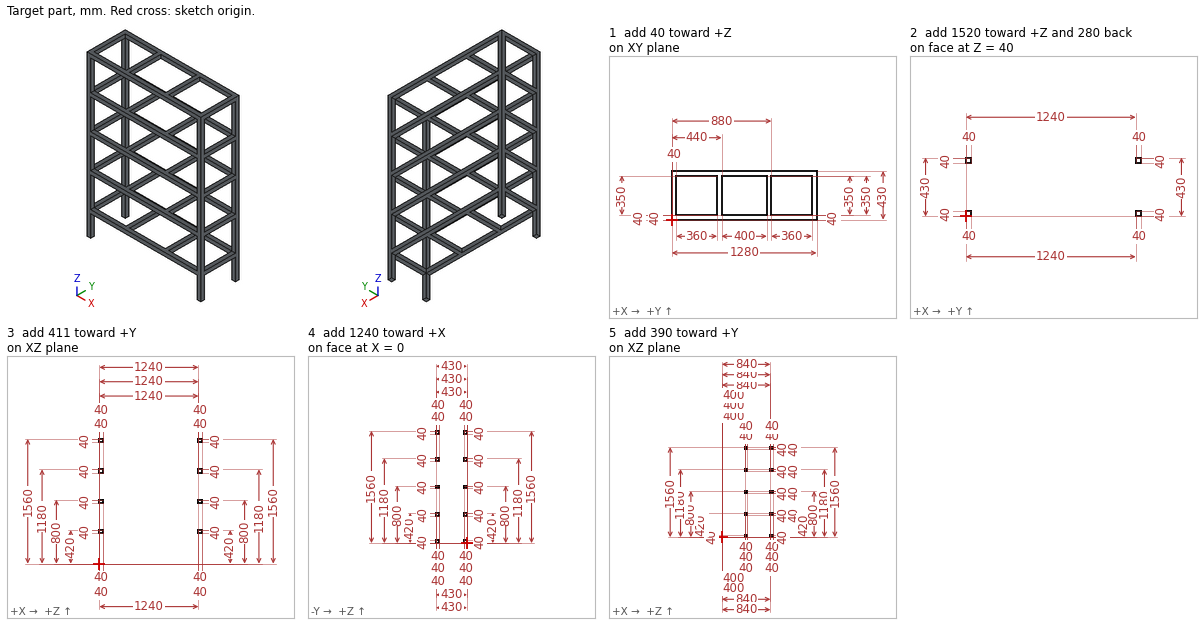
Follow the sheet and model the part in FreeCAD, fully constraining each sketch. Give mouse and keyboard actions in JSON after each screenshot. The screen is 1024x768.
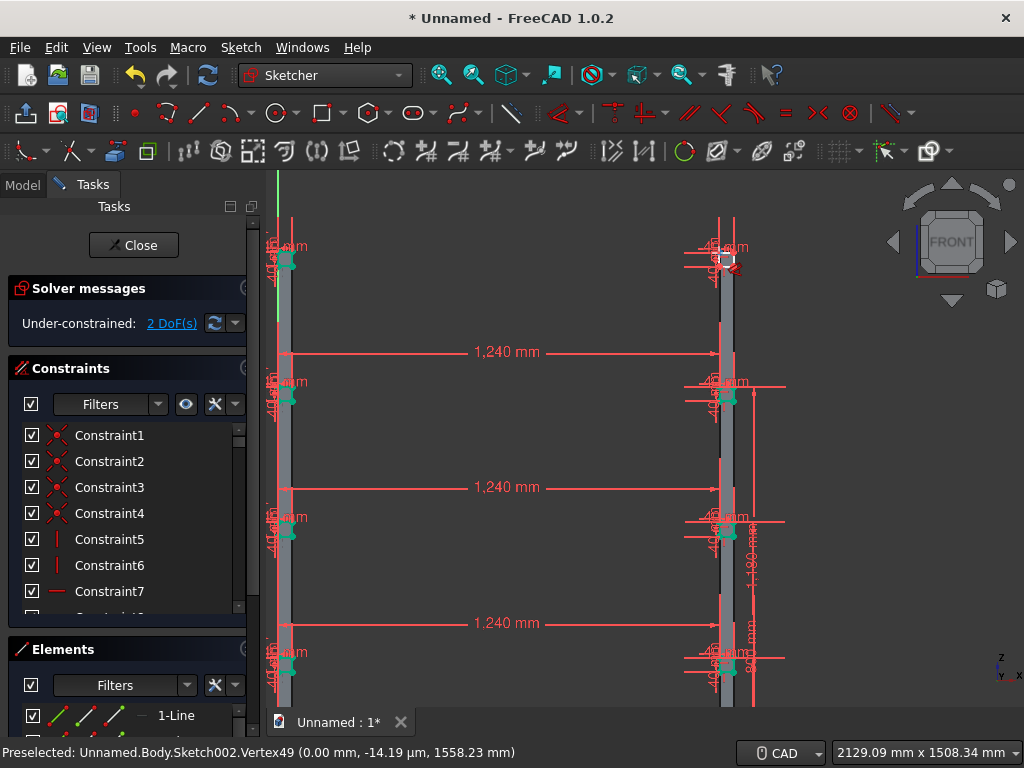
{"action": "left_click", "coordinate": [719, 253]}
{"action": "left_click", "coordinate": [507, 219]}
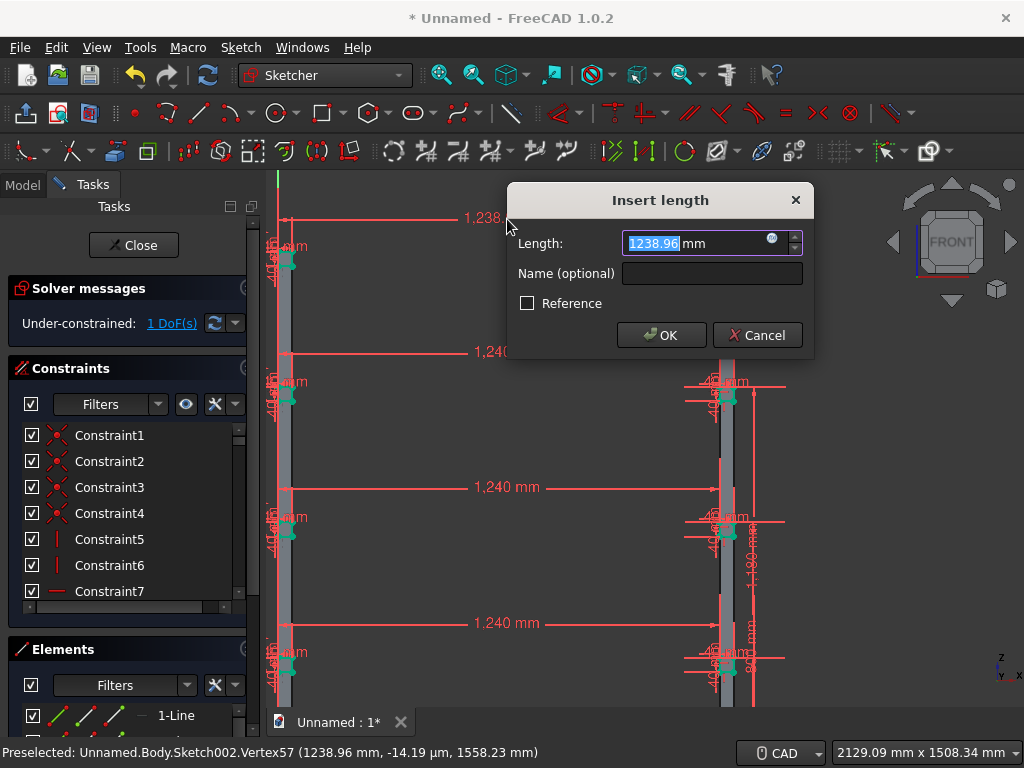
{"action": "type", "text": "1240"}
{"action": "key", "text": "Return"}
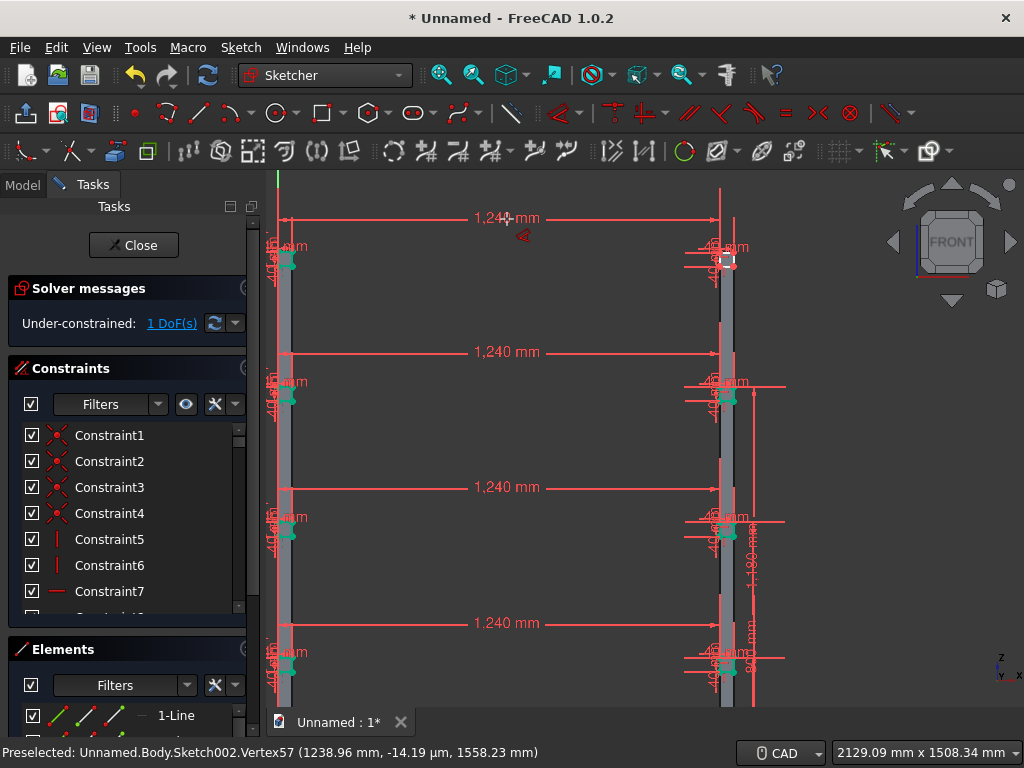
{"action": "left_click", "coordinate": [720, 253]}
{"action": "left_click", "coordinate": [754, 466]}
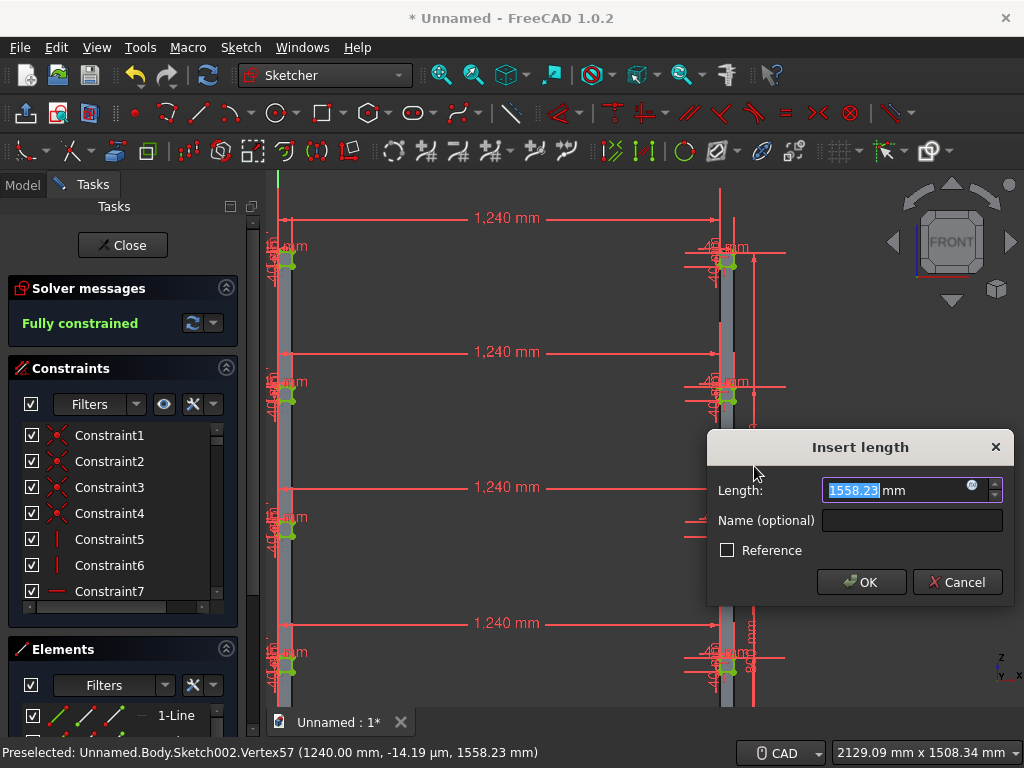
{"action": "type", "text": "1560"}
{"action": "key", "text": "Return"}
{"action": "key", "text": "Escape"}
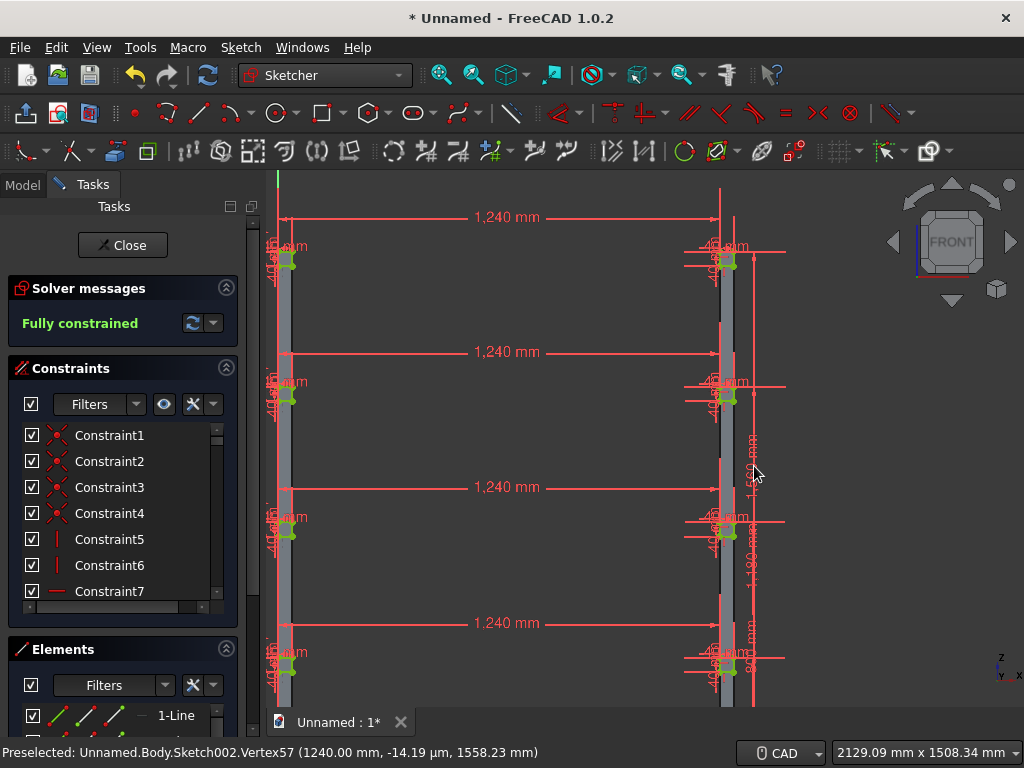
{"action": "left_click", "coordinate": [123, 245]}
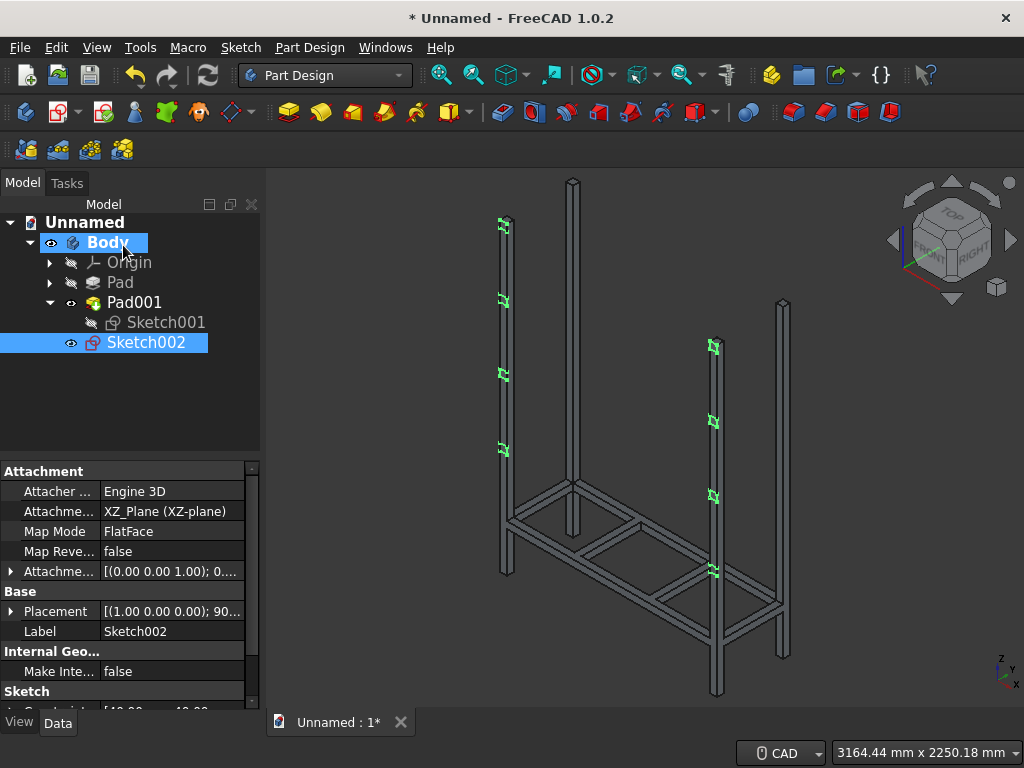
{"action": "left_click", "coordinate": [290, 112]}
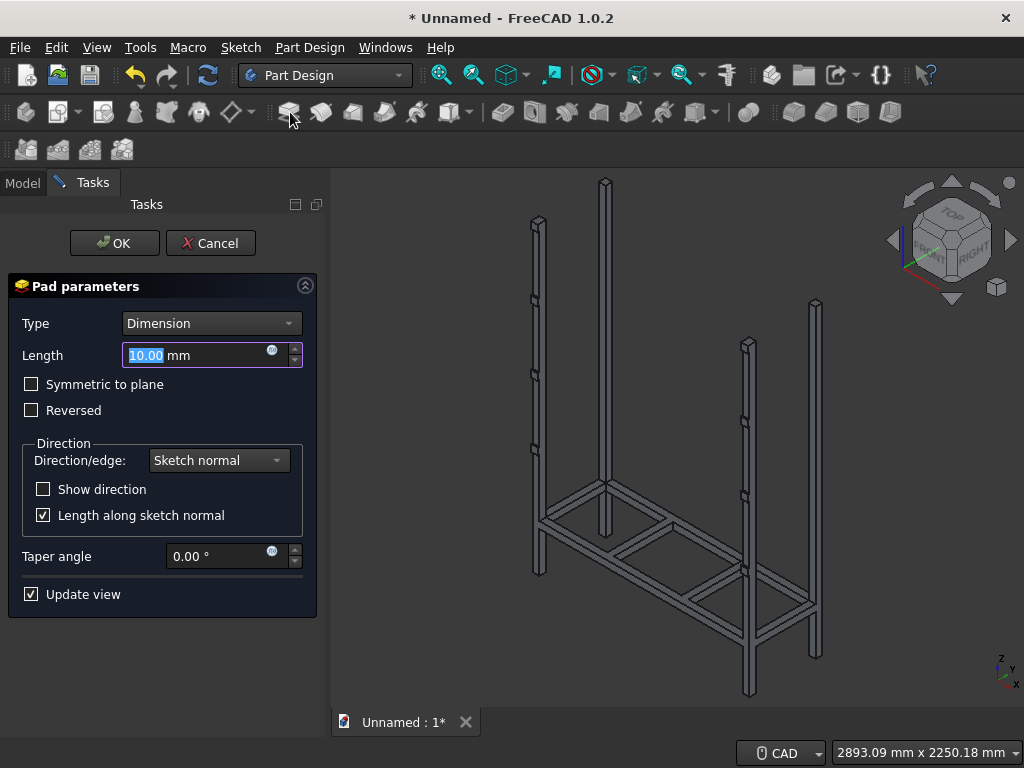
{"action": "type", "text": "411"}
{"action": "key", "text": "Tab"}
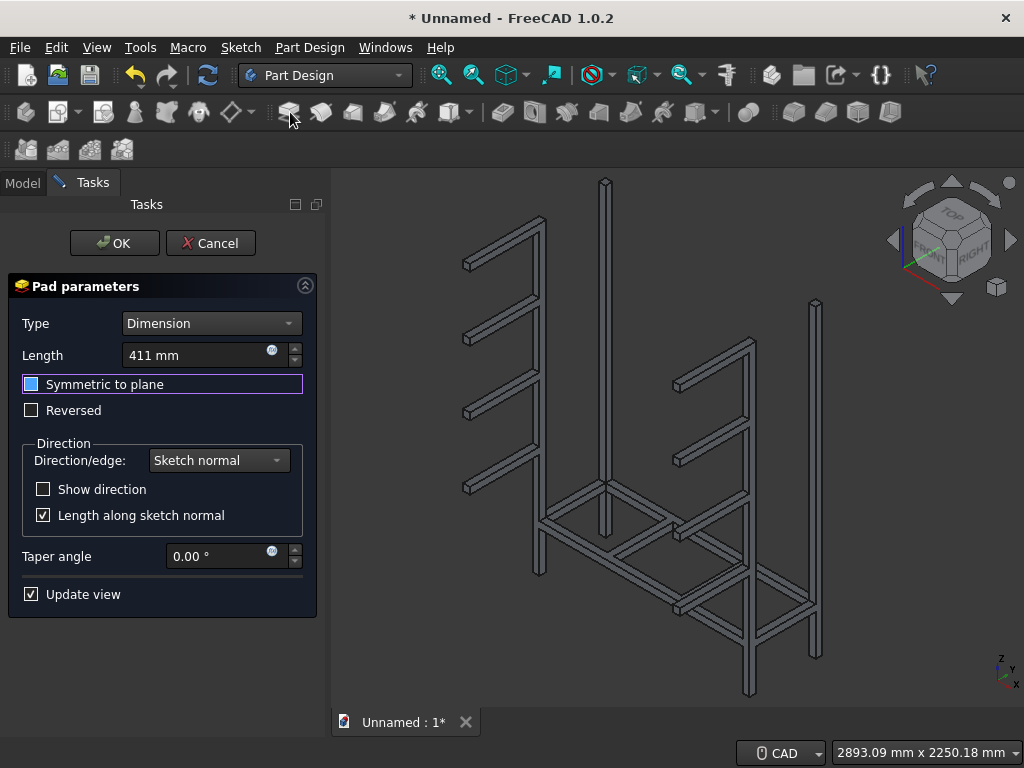
{"action": "left_click", "coordinate": [30, 410]}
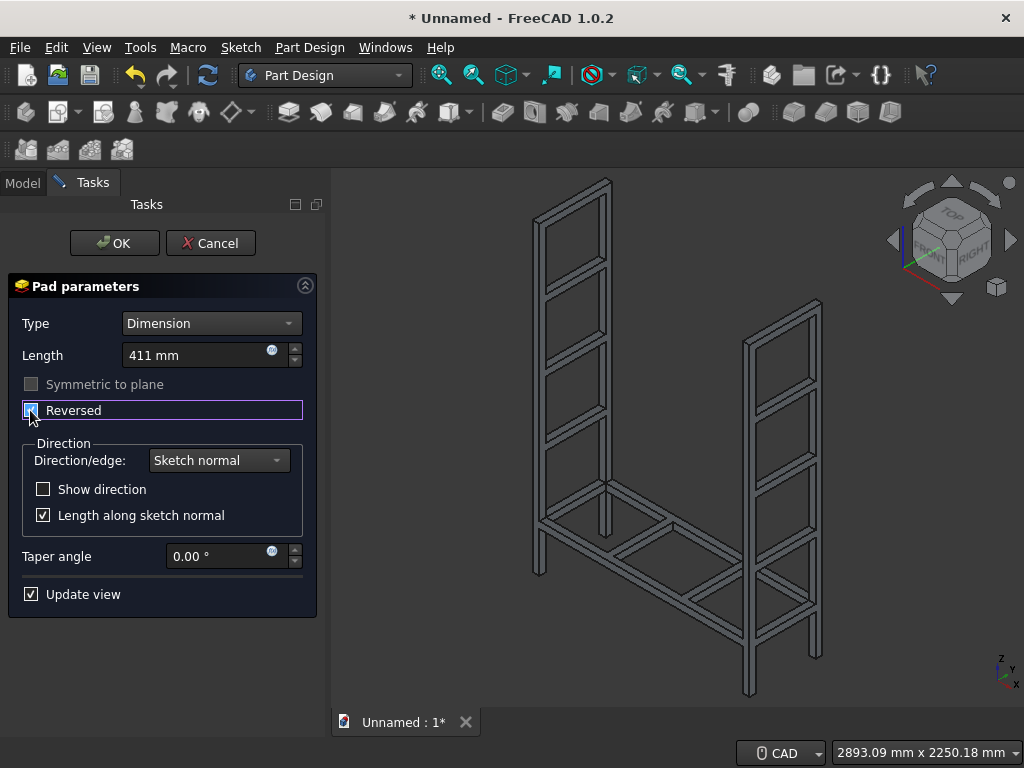
{"action": "left_click", "coordinate": [115, 243]}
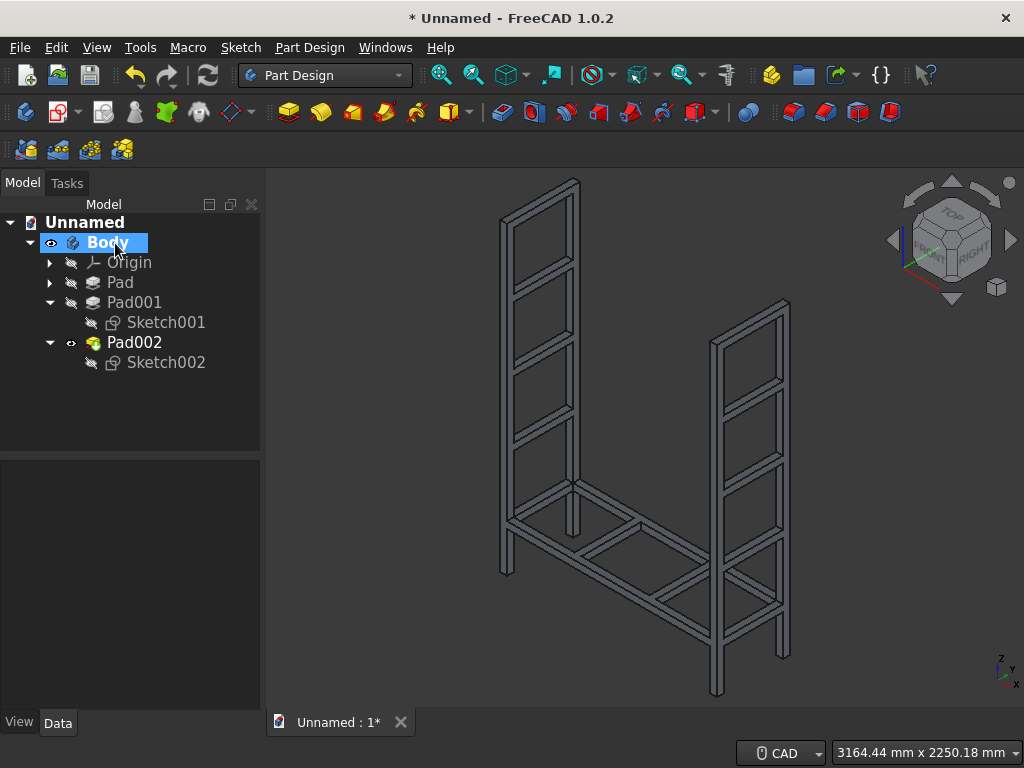
{"action": "key", "text": "6"}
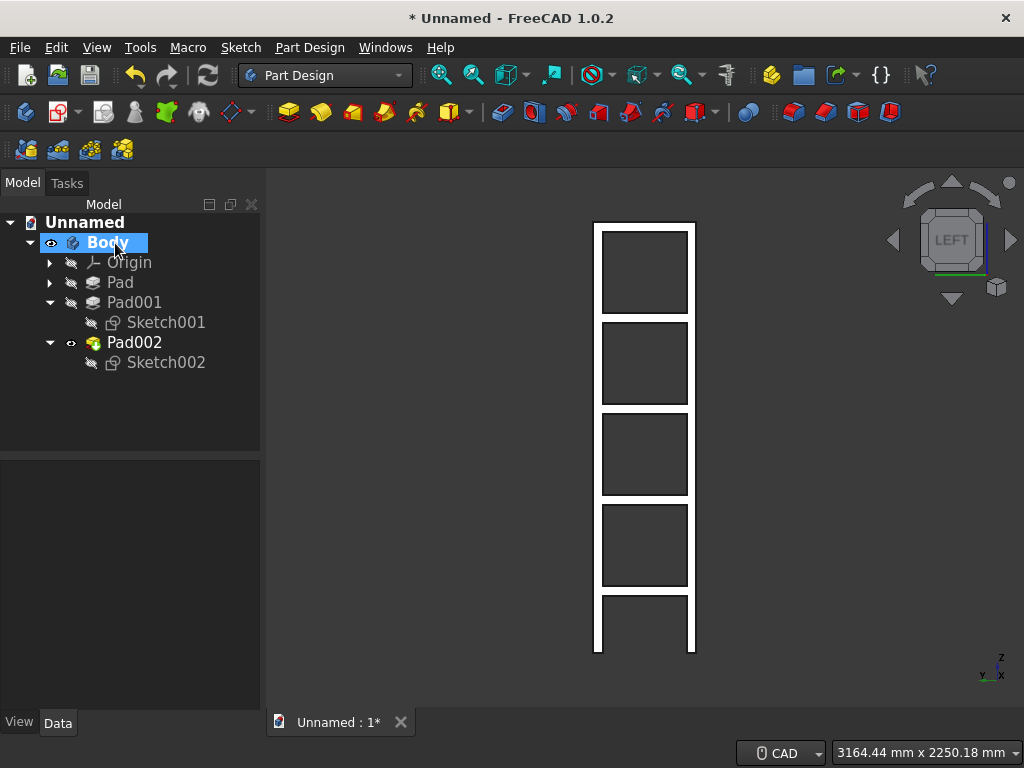
{"action": "scroll", "coordinate": [689, 498], "scroll_direction": "up", "scroll_amount": 5}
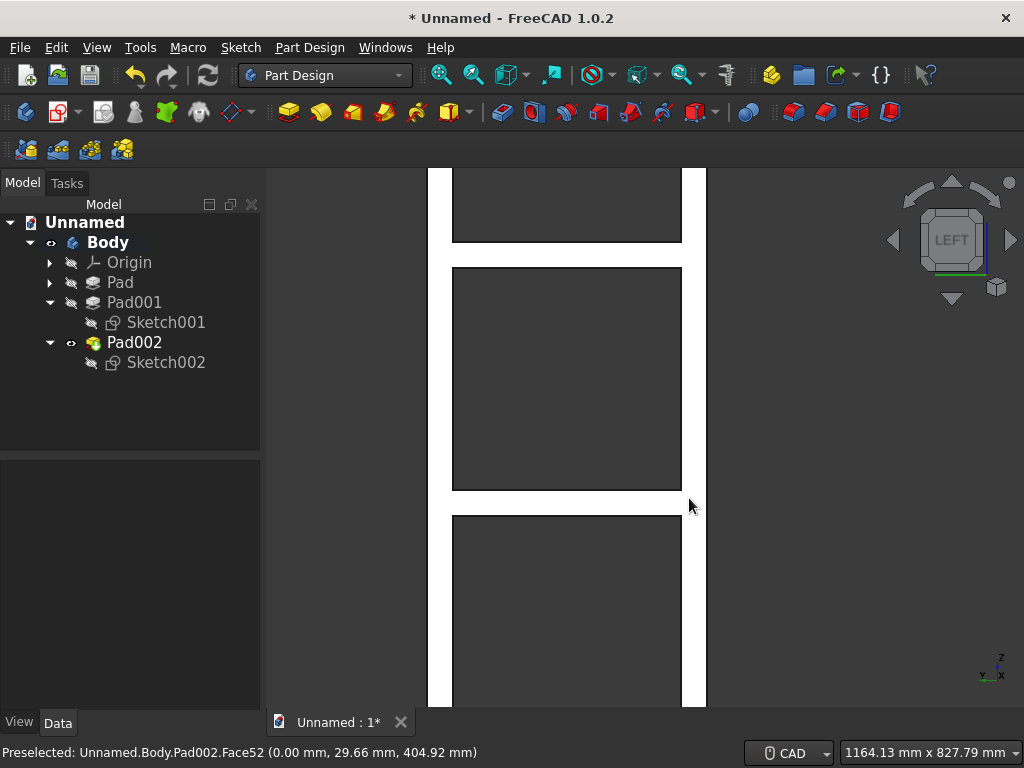
{"action": "left_click", "coordinate": [687, 500]}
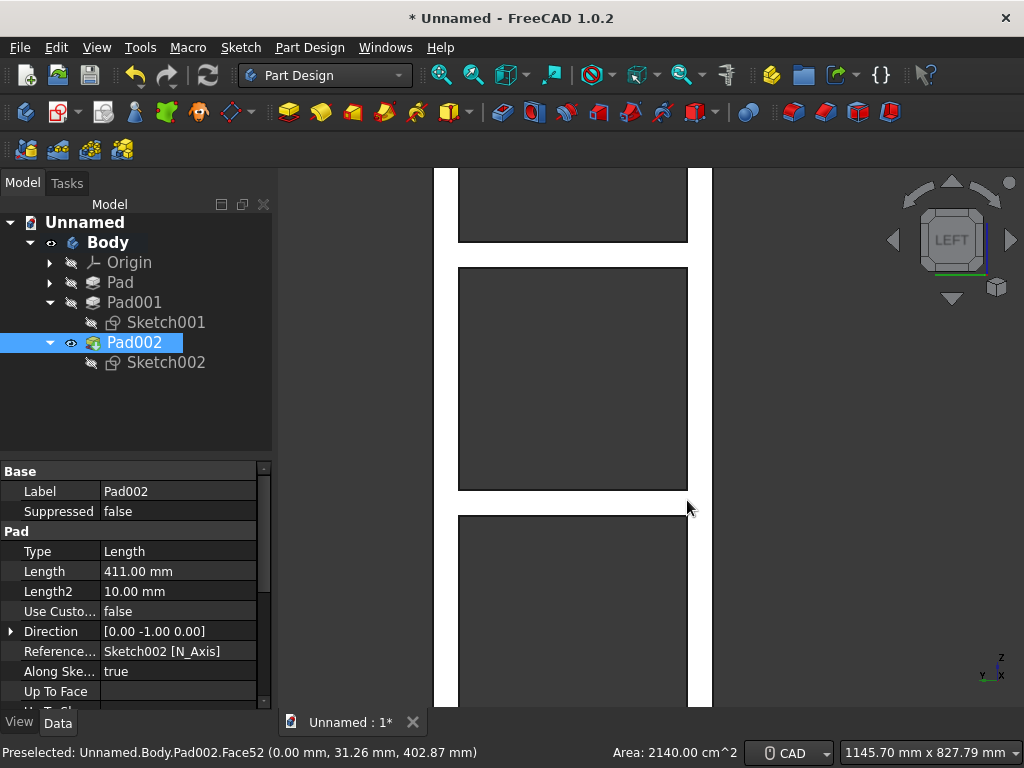
{"action": "left_click", "coordinate": [58, 112]}